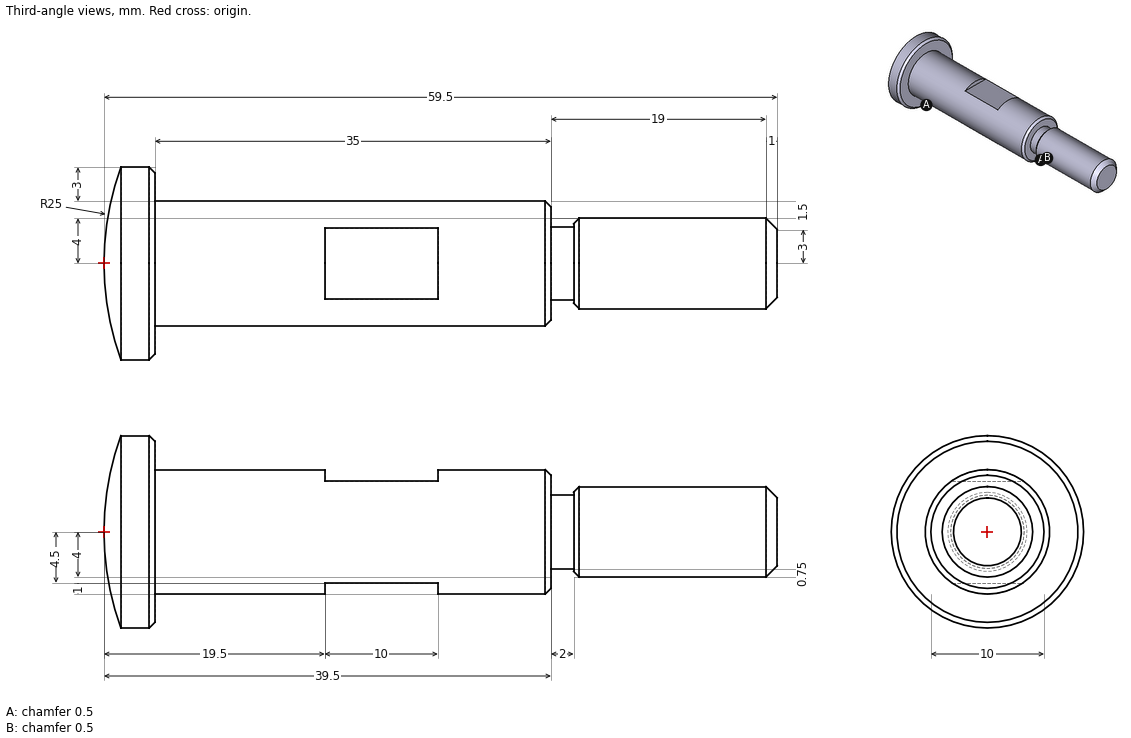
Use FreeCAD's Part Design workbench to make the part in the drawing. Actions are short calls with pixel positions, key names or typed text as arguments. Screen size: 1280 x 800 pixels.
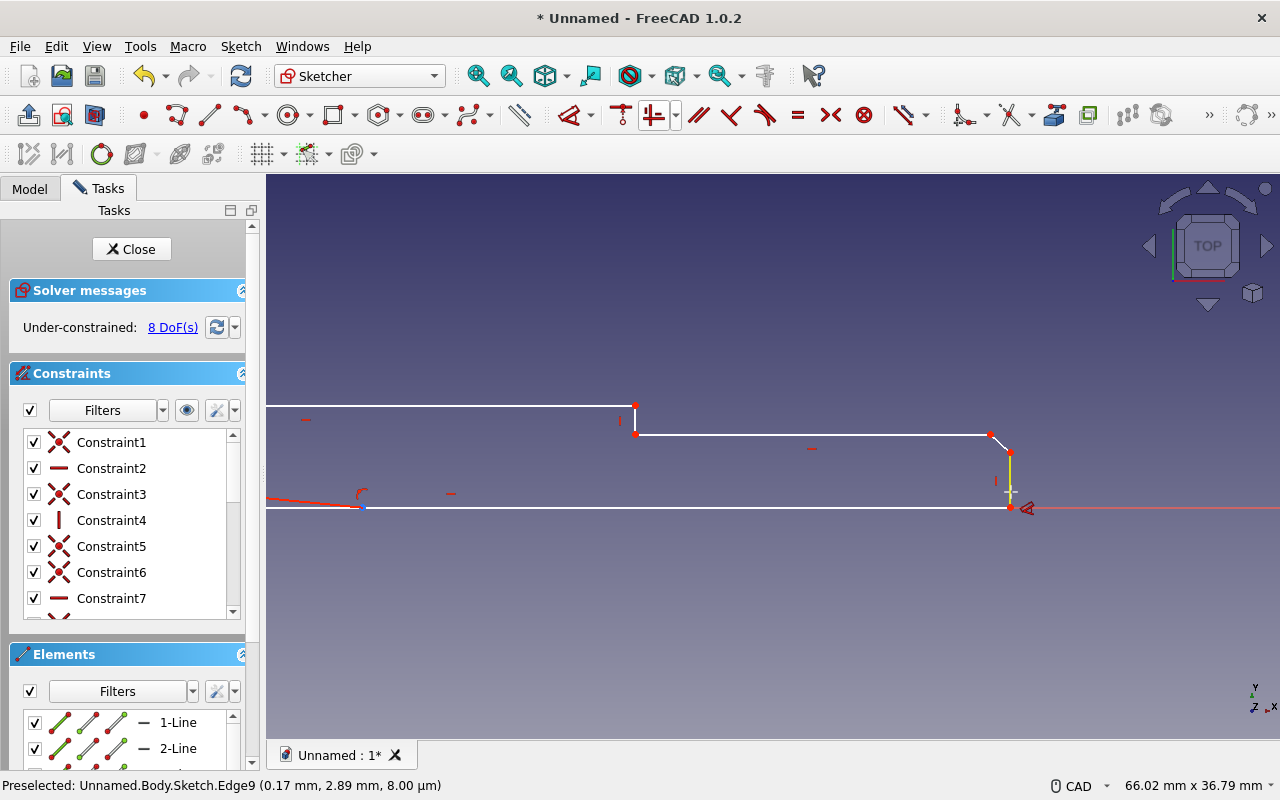
click(1010, 491)
click(1044, 480)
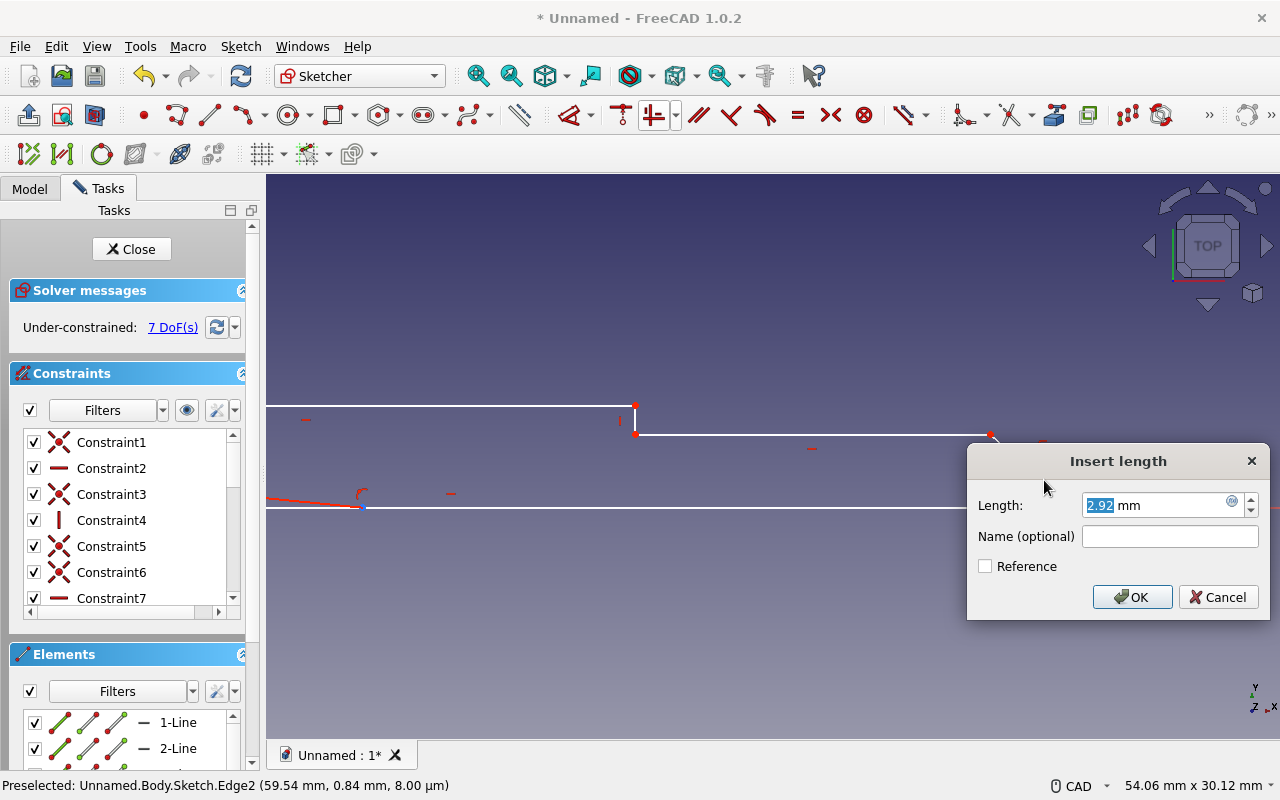
text(3)
key(Return)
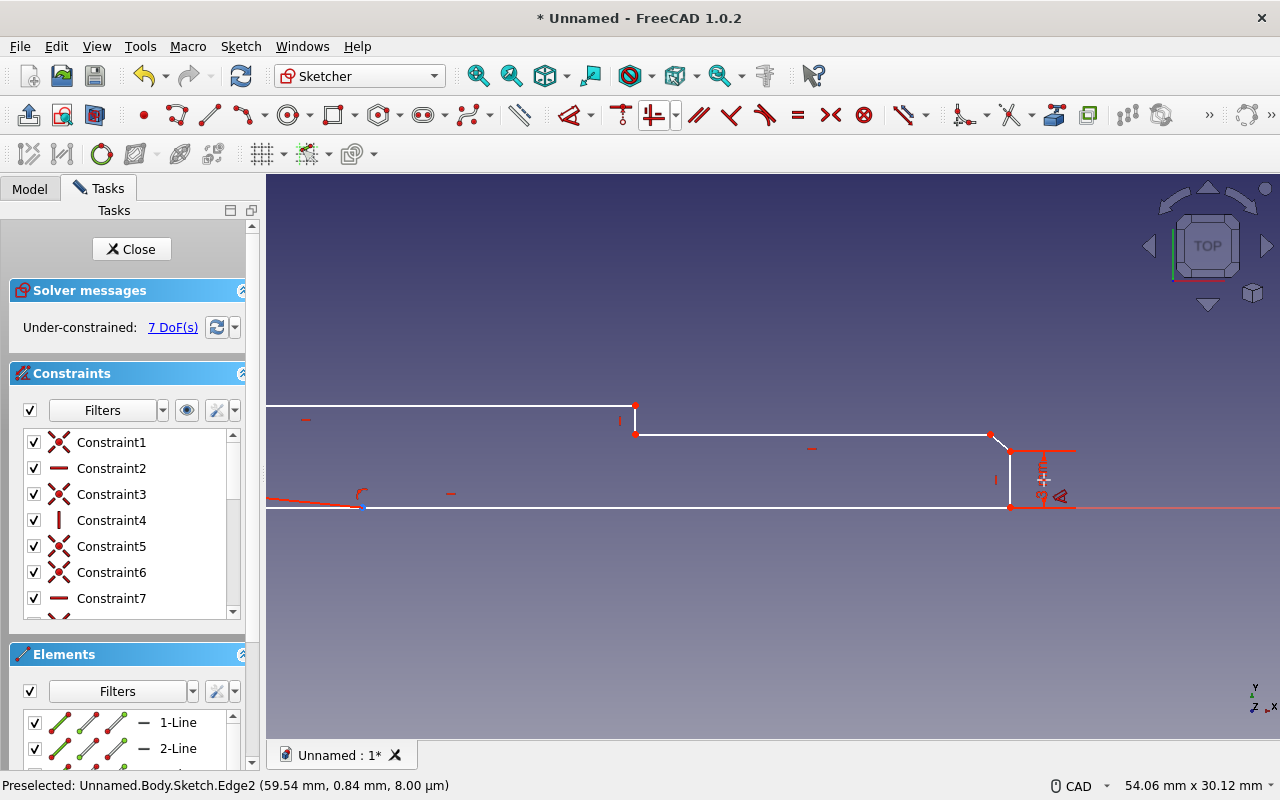
scroll(1012, 491, down, 3)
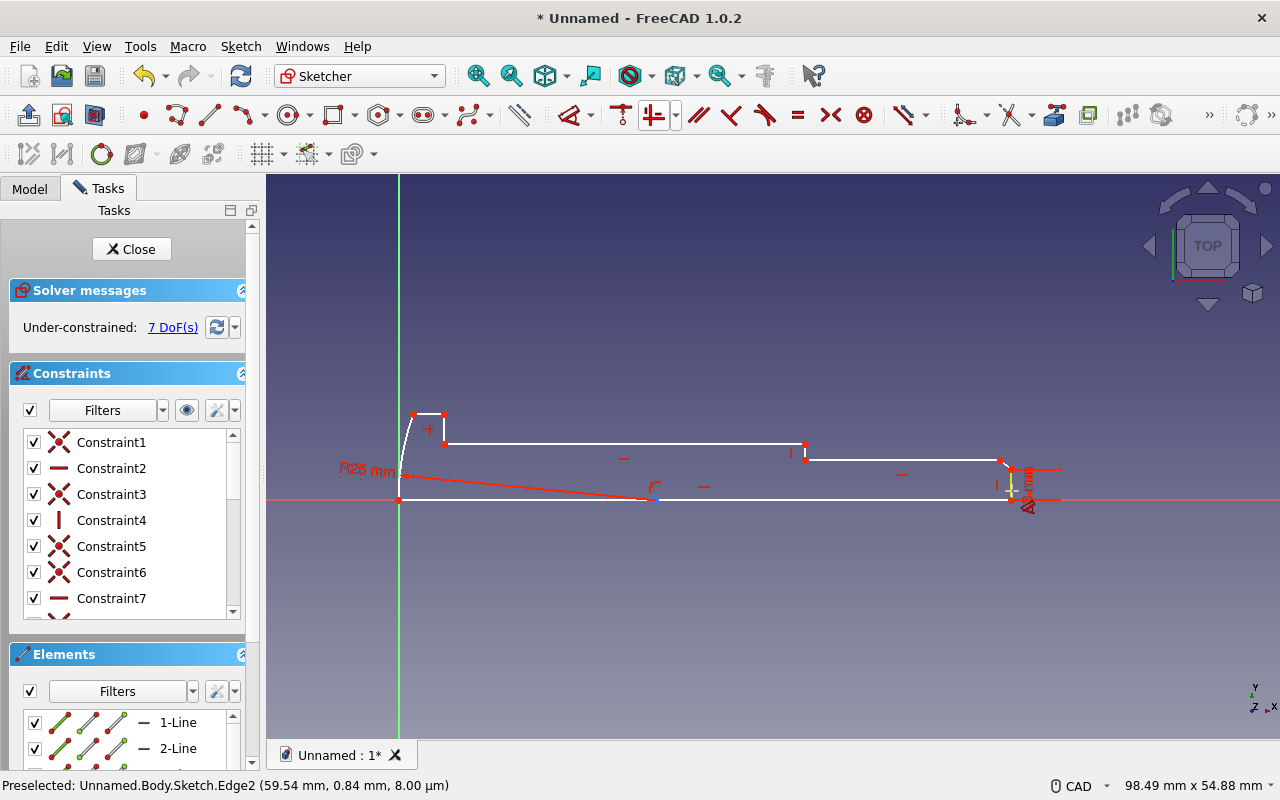
scroll(444, 435, up, 3)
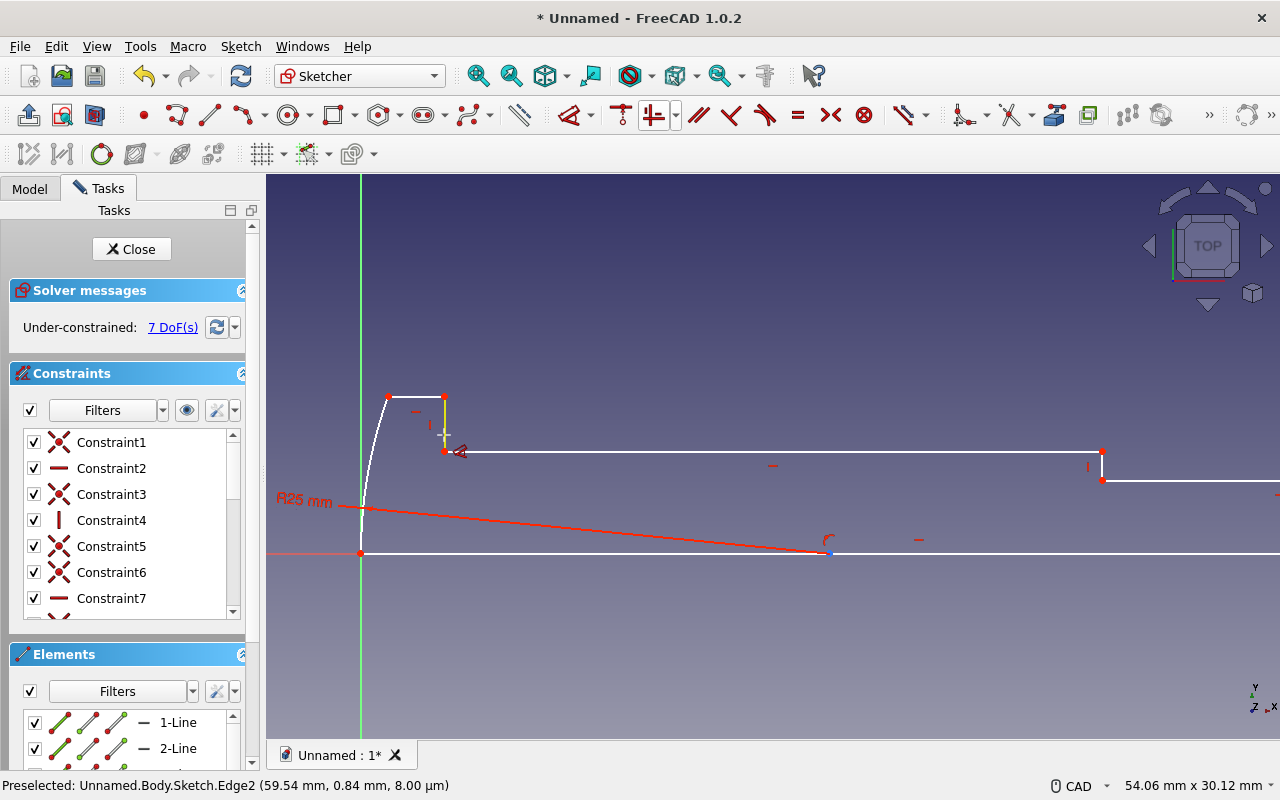
click(445, 435)
click(411, 424)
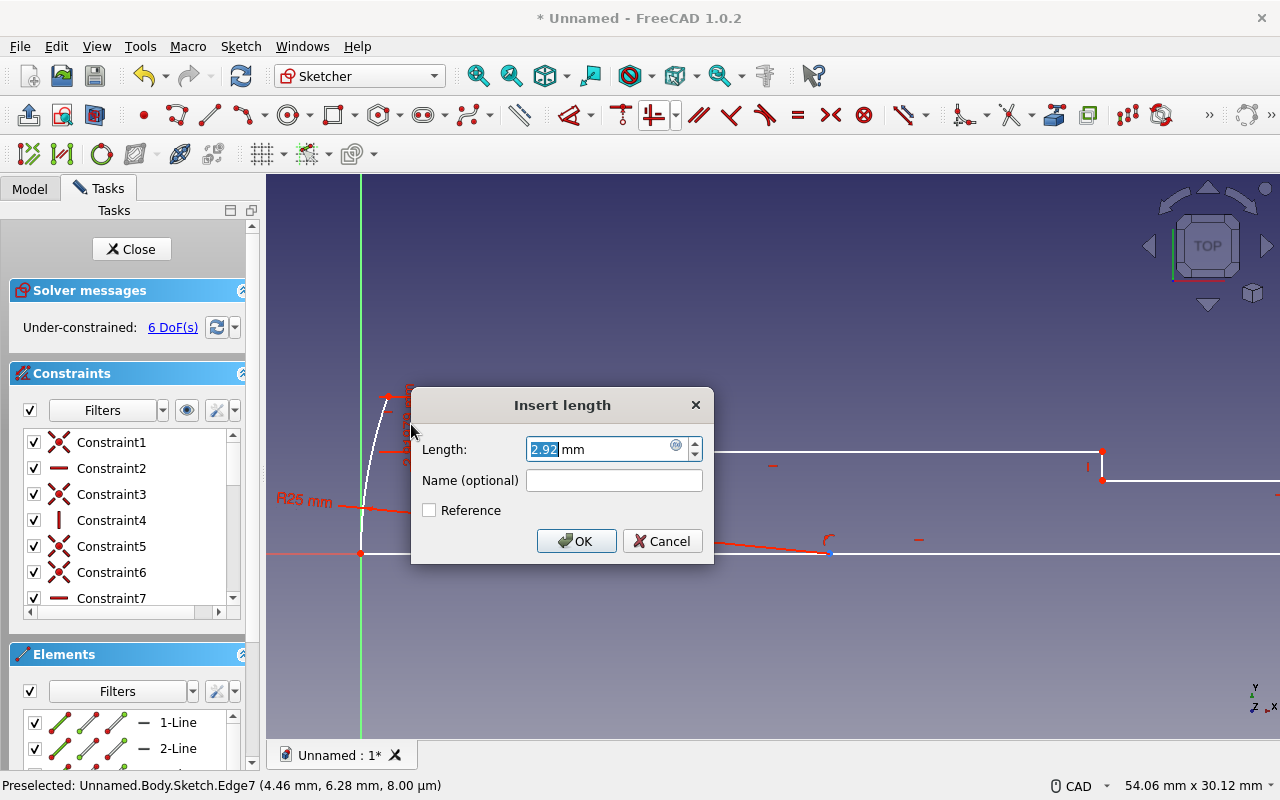
text(3)
key(Return)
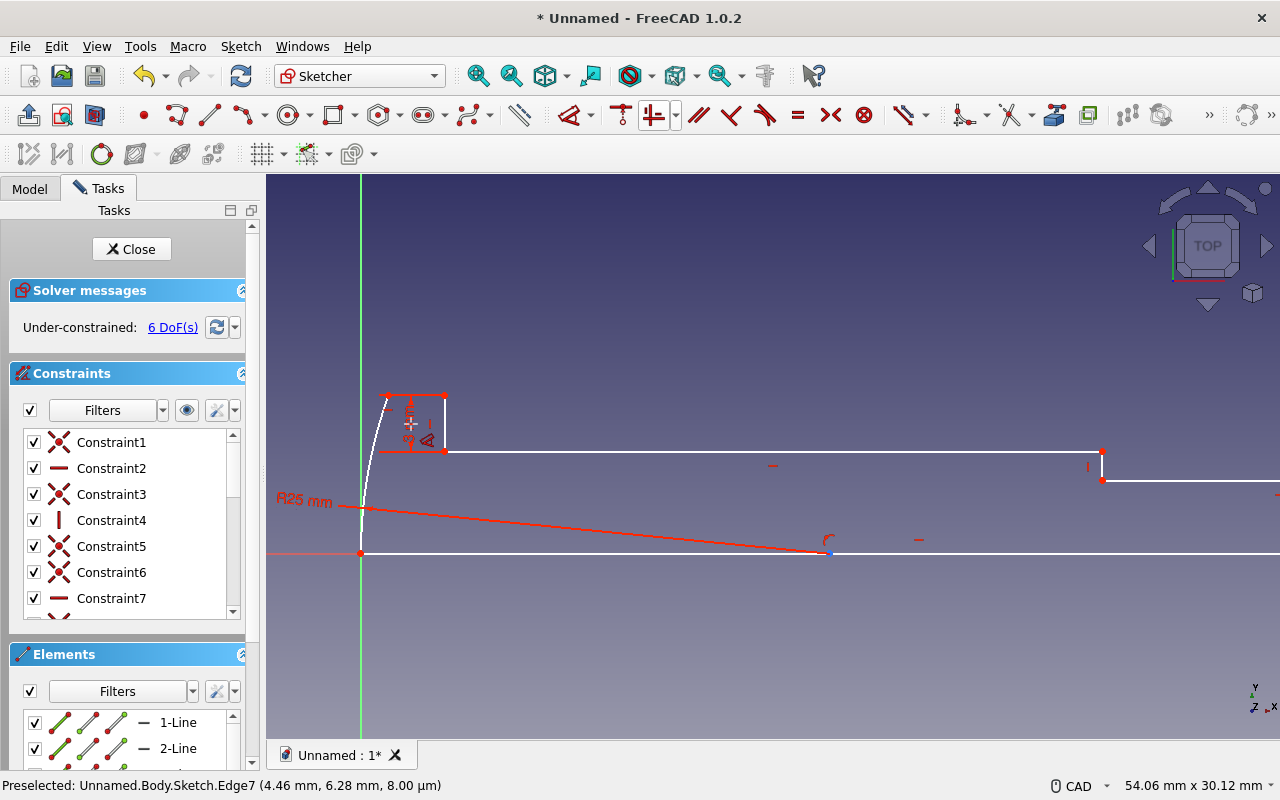
scroll(444, 435, down, 3)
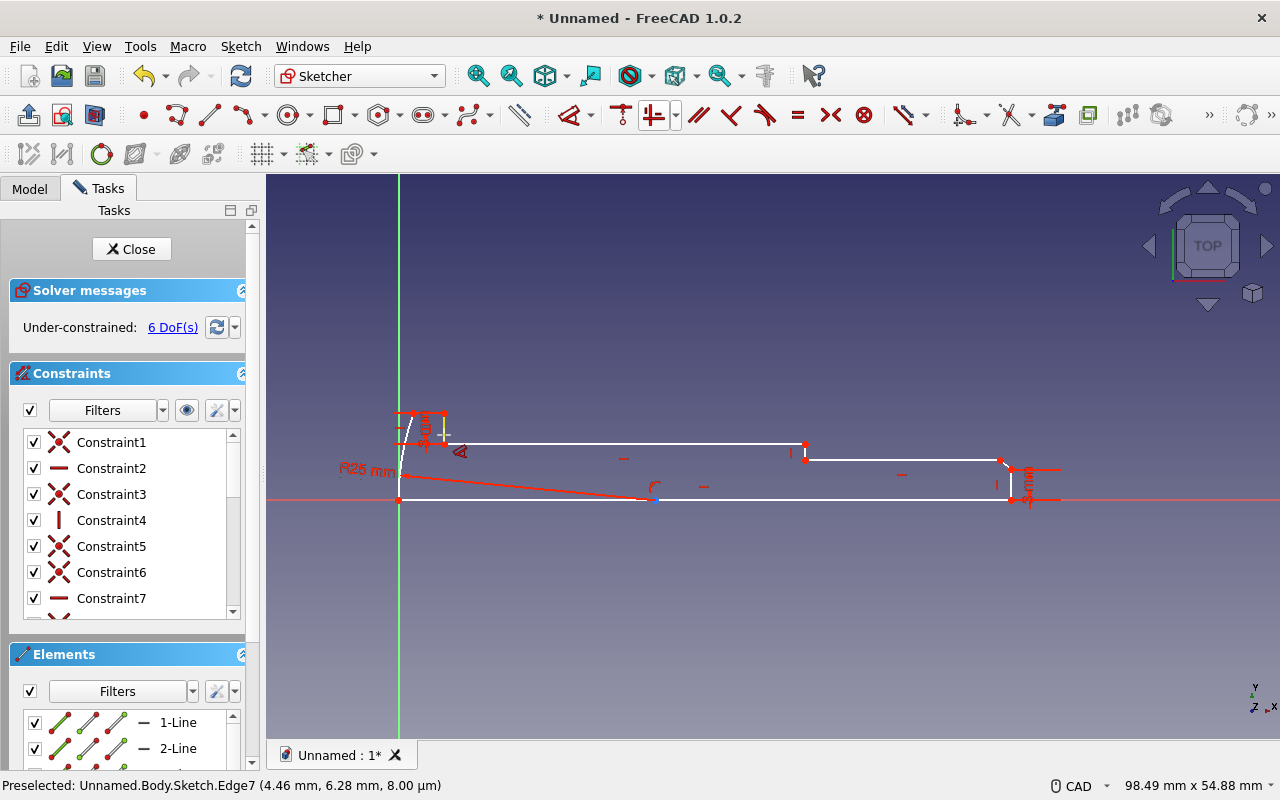
click(942, 460)
click(903, 426)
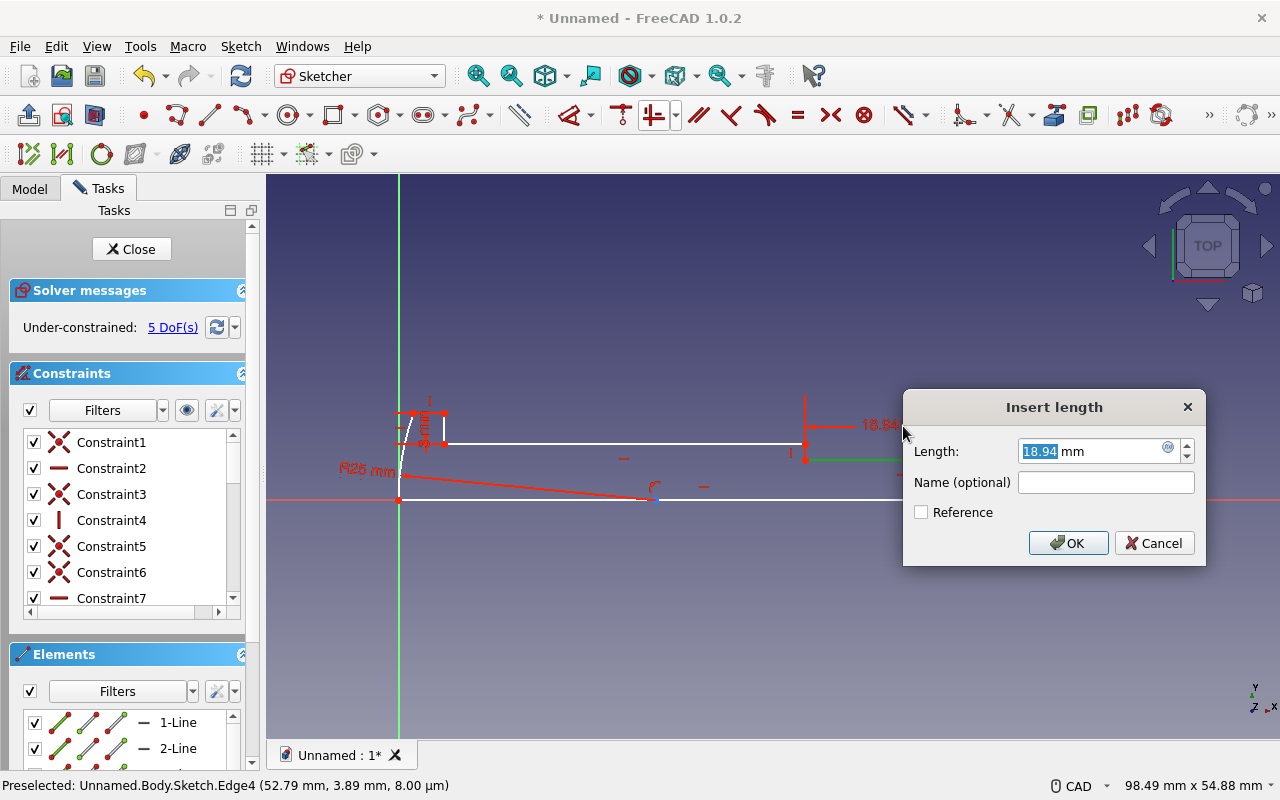
text(19)
key(Return)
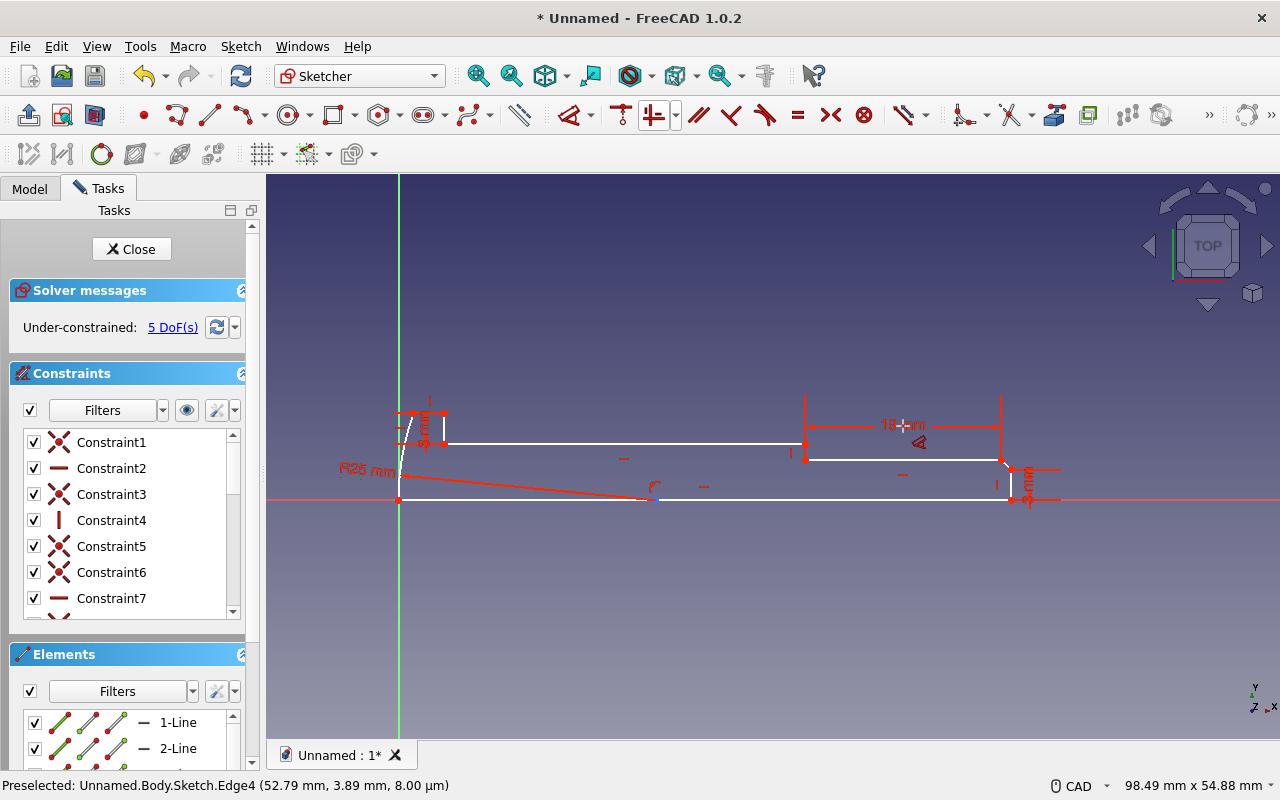
click(697, 444)
click(625, 410)